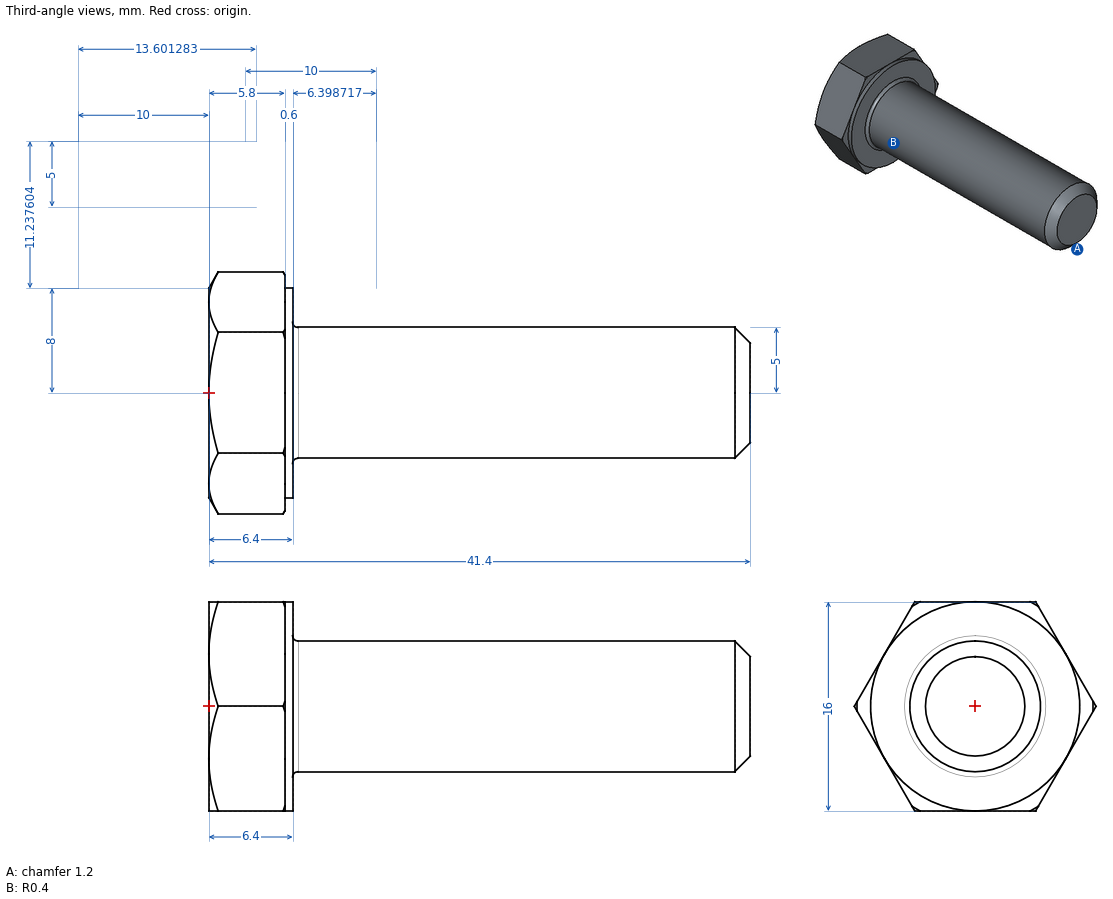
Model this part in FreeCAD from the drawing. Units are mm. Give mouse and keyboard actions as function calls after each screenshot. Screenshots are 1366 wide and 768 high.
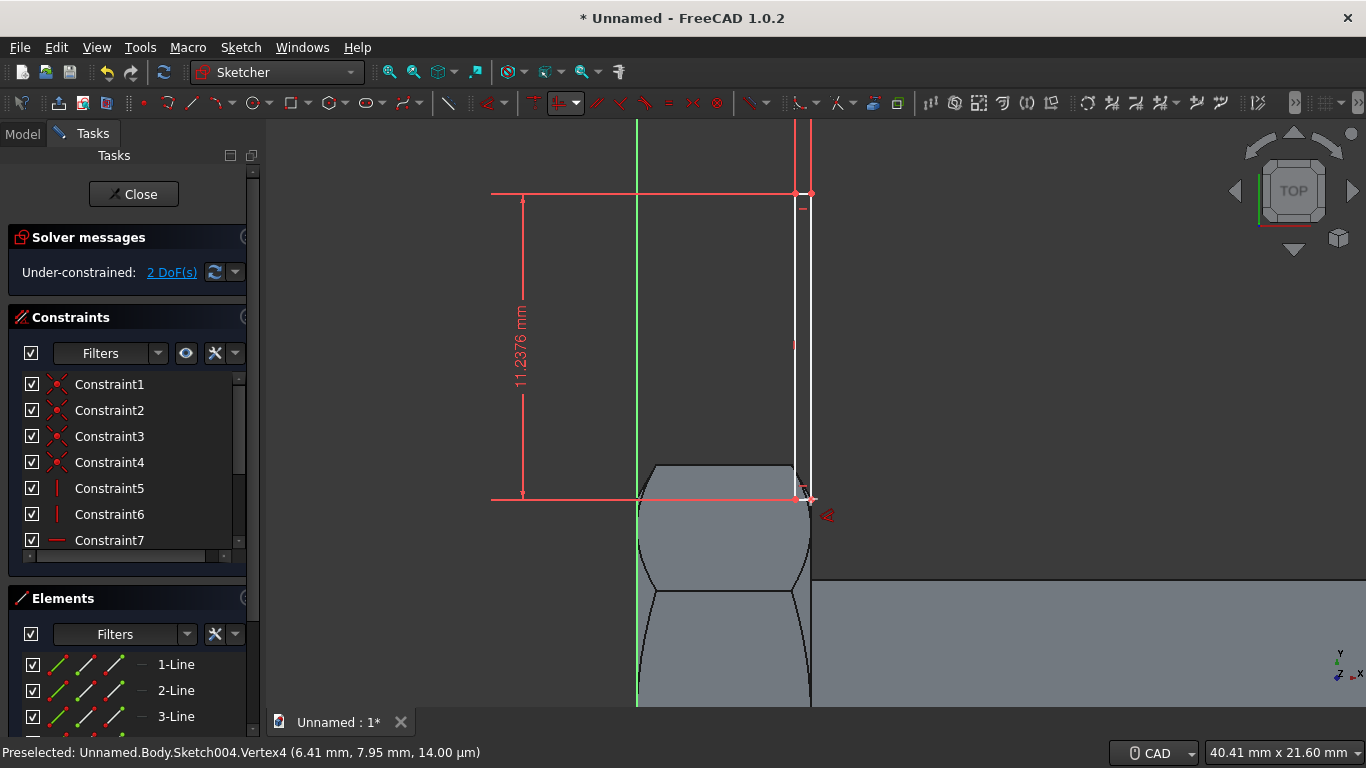
click(795, 500)
click(603, 589)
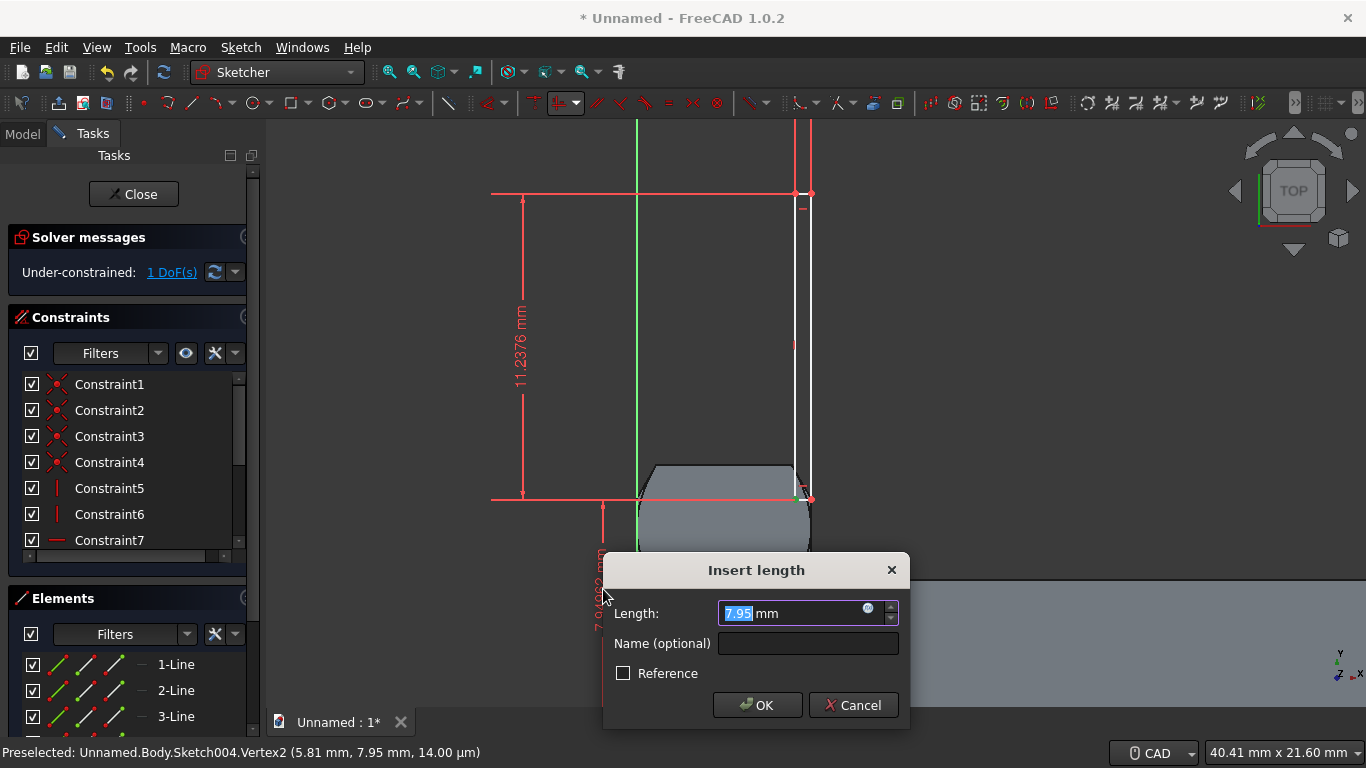
text(8)
key(Return)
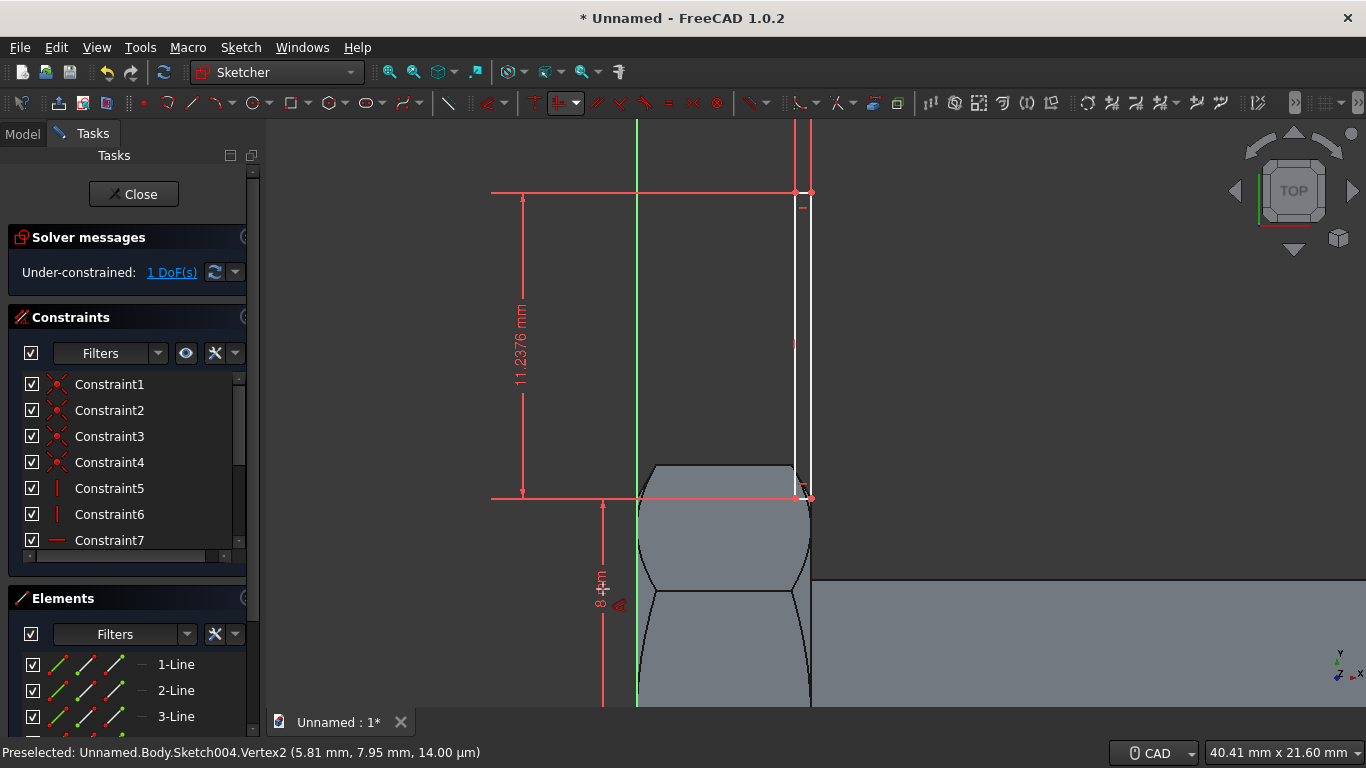
click(795, 193)
click(716, 159)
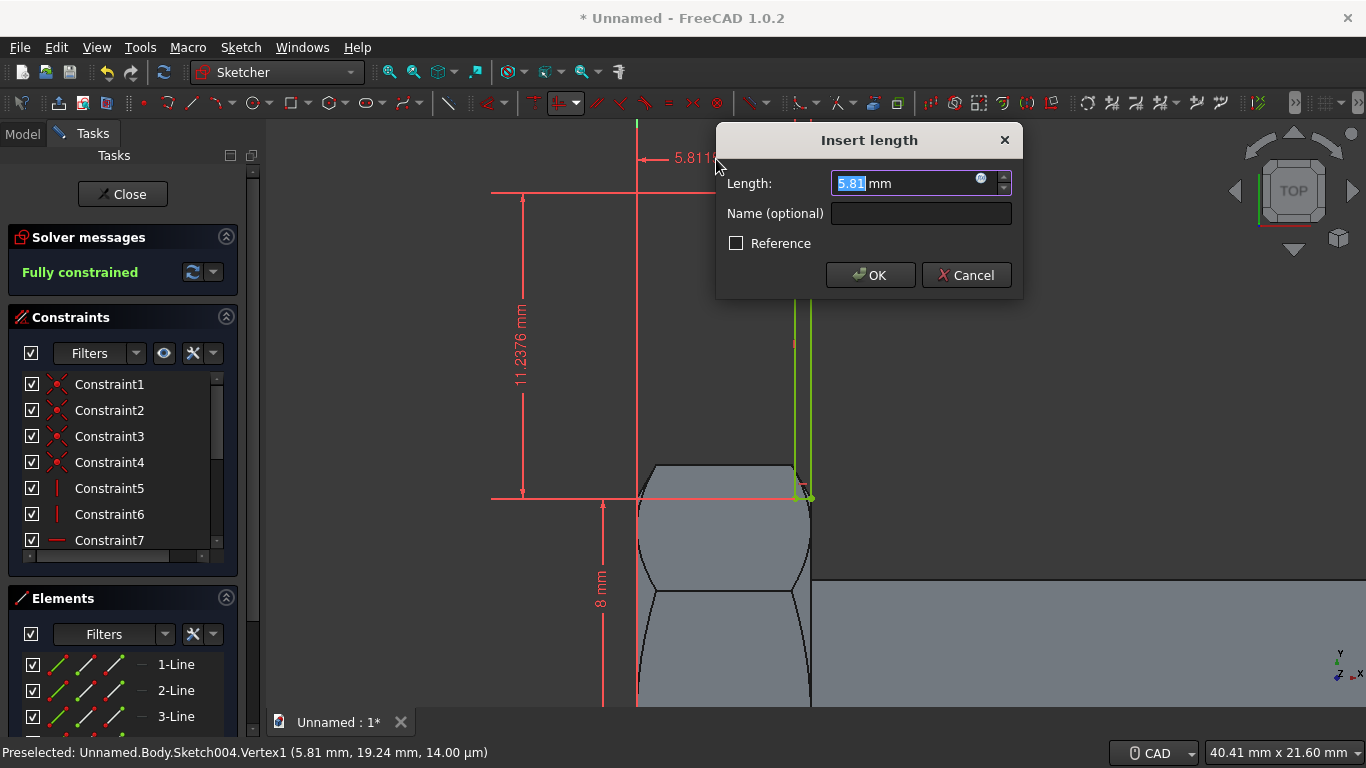
text(5.8)
key(Return)
key(Escape)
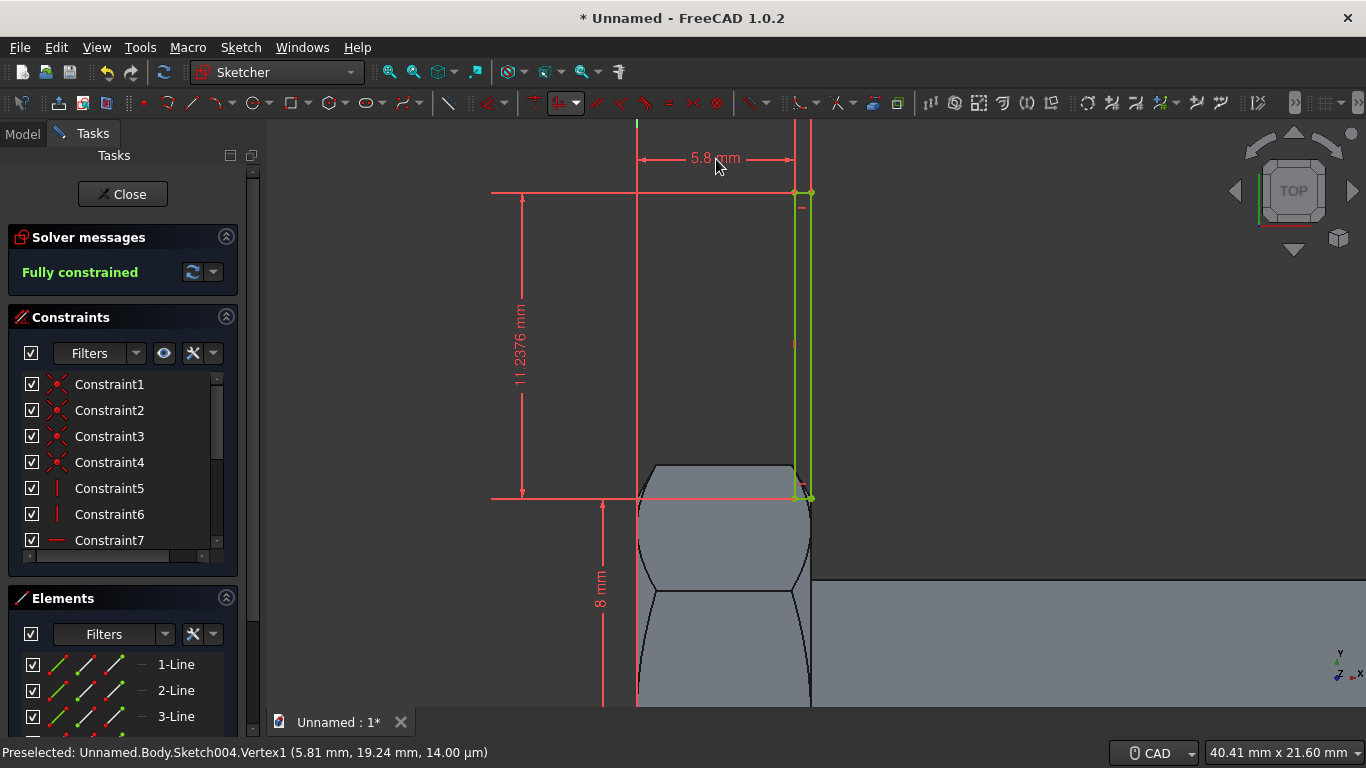
click(123, 194)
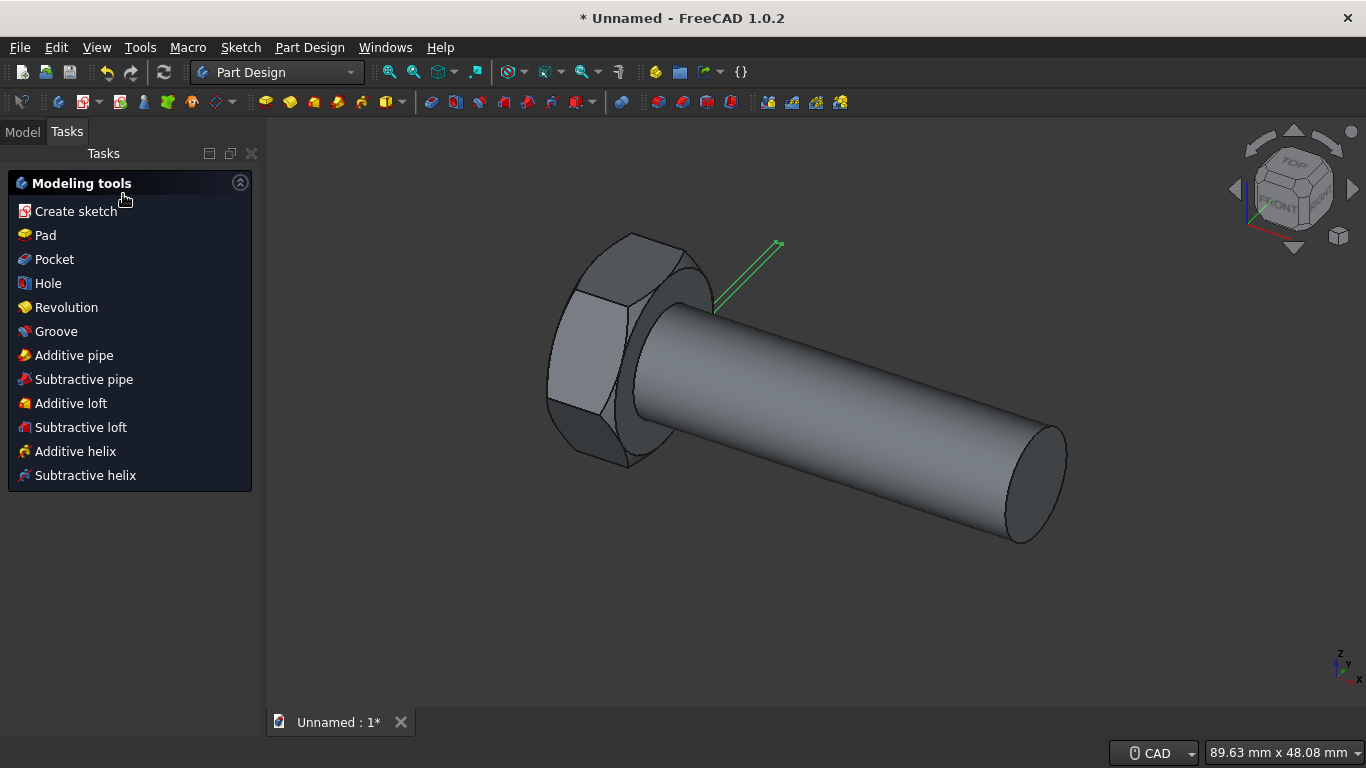
click(480, 102)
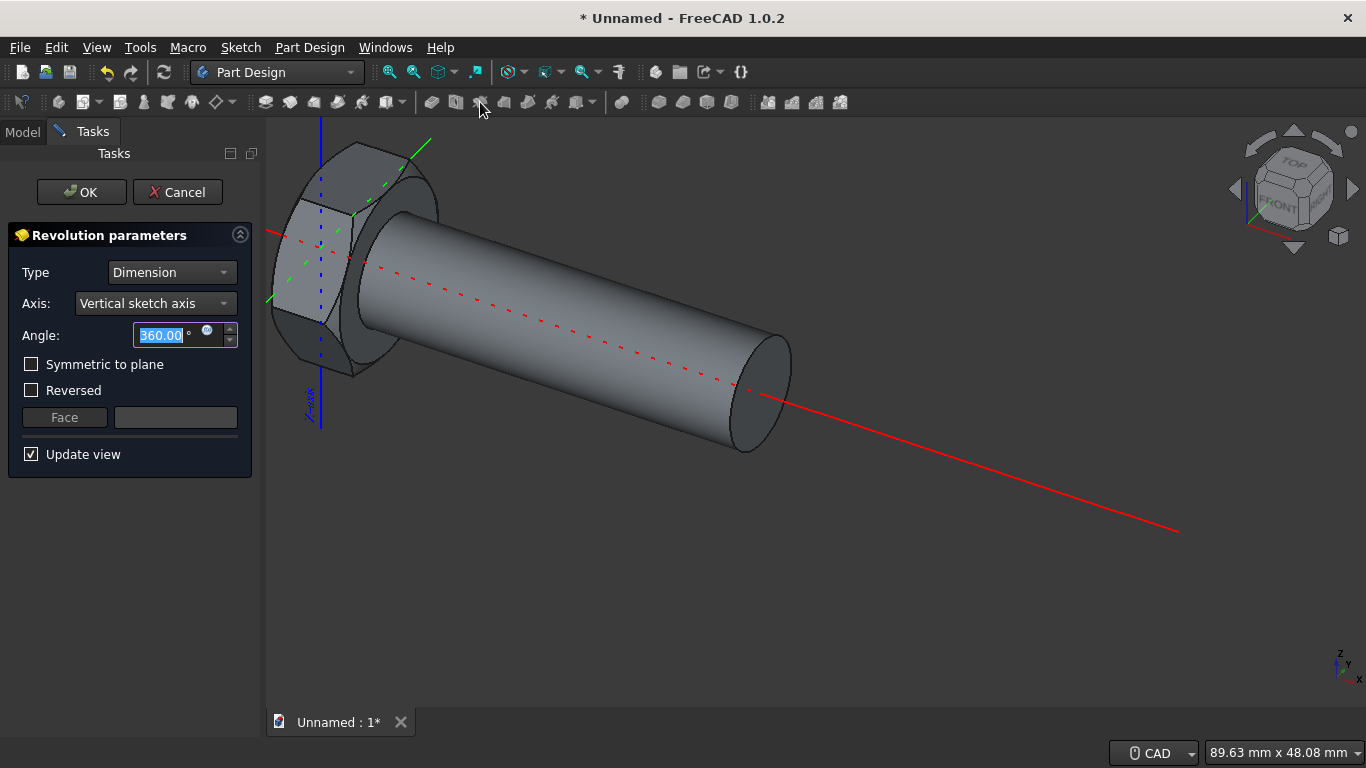
click(156, 304)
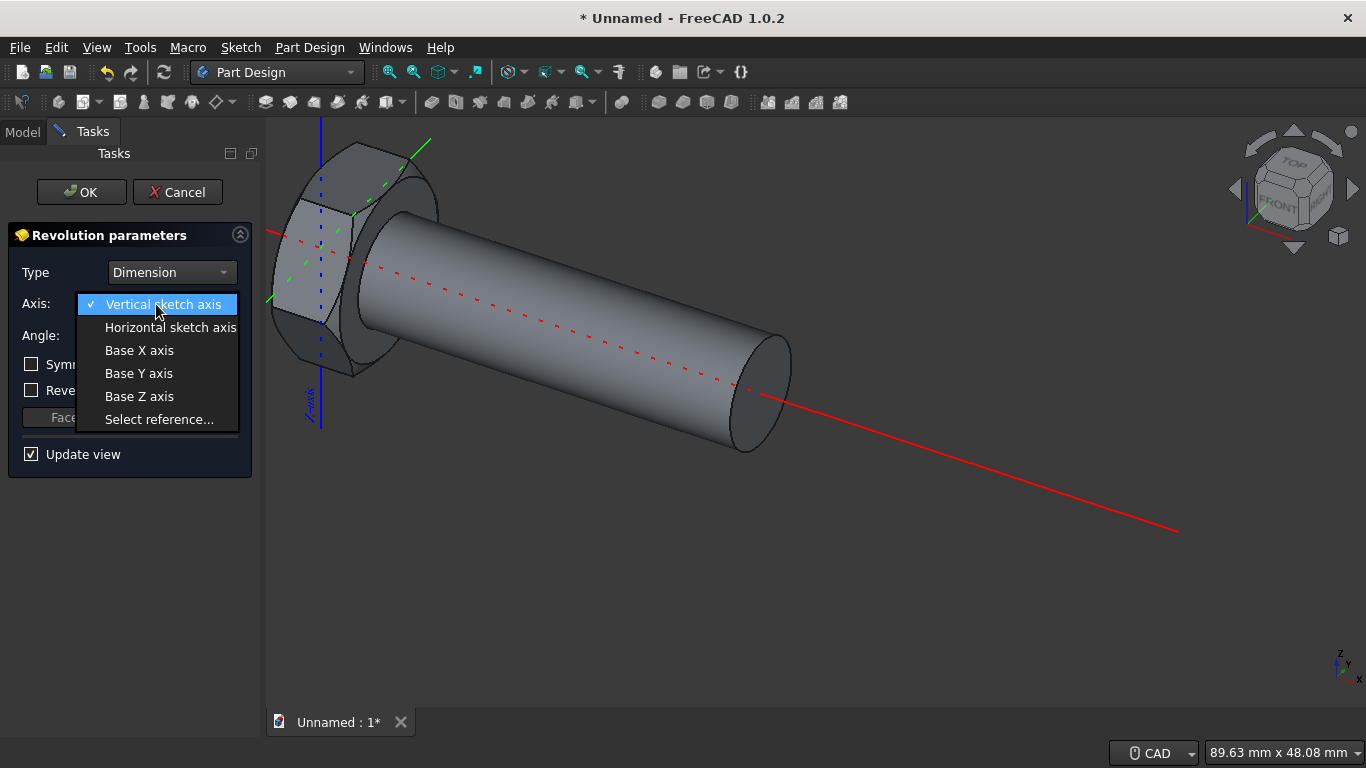
click(156, 328)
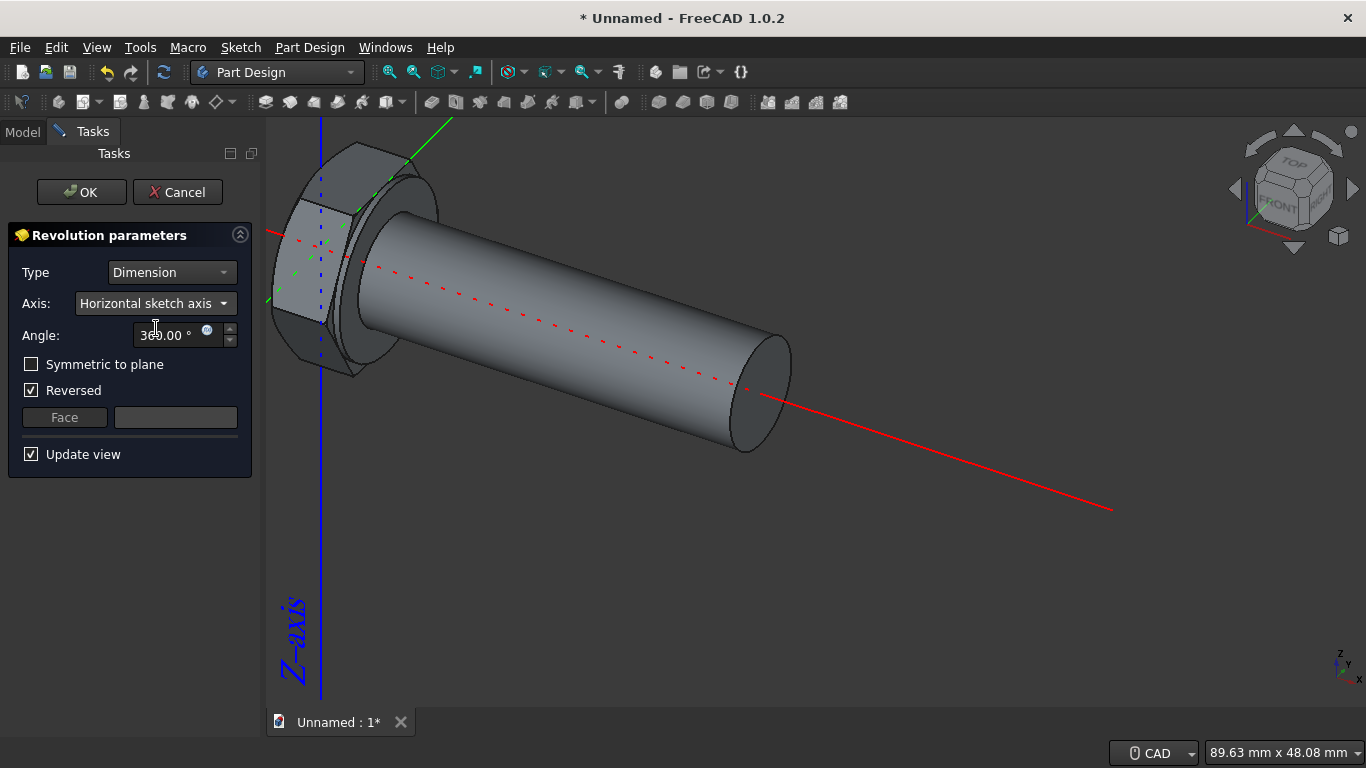
click(82, 192)